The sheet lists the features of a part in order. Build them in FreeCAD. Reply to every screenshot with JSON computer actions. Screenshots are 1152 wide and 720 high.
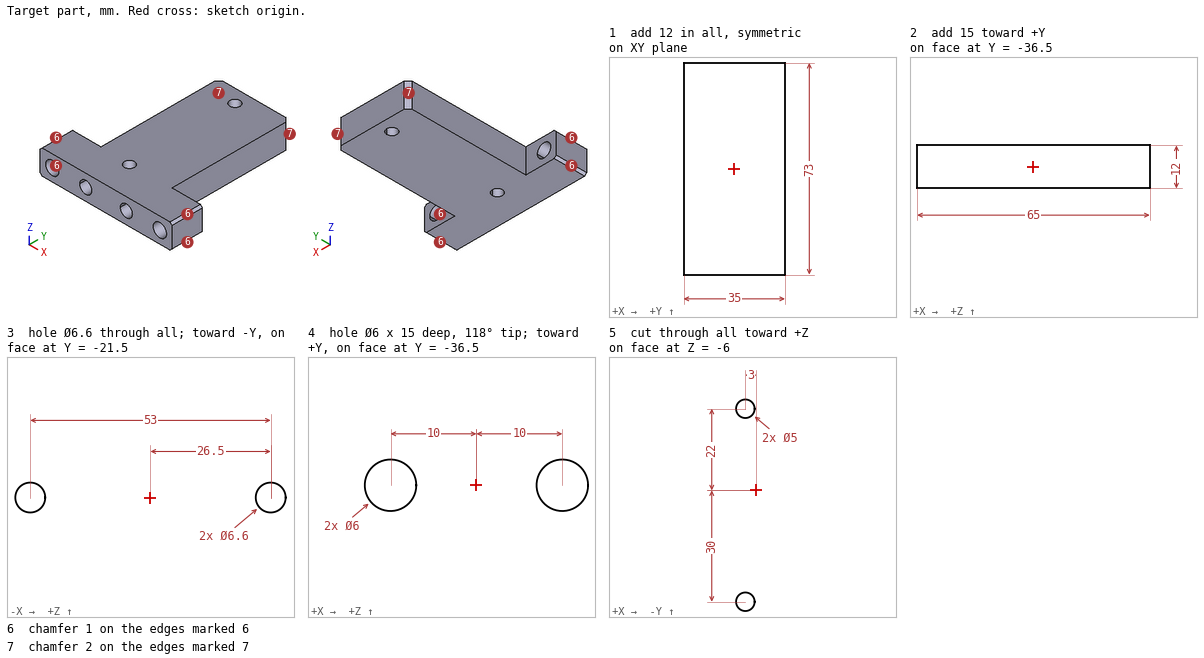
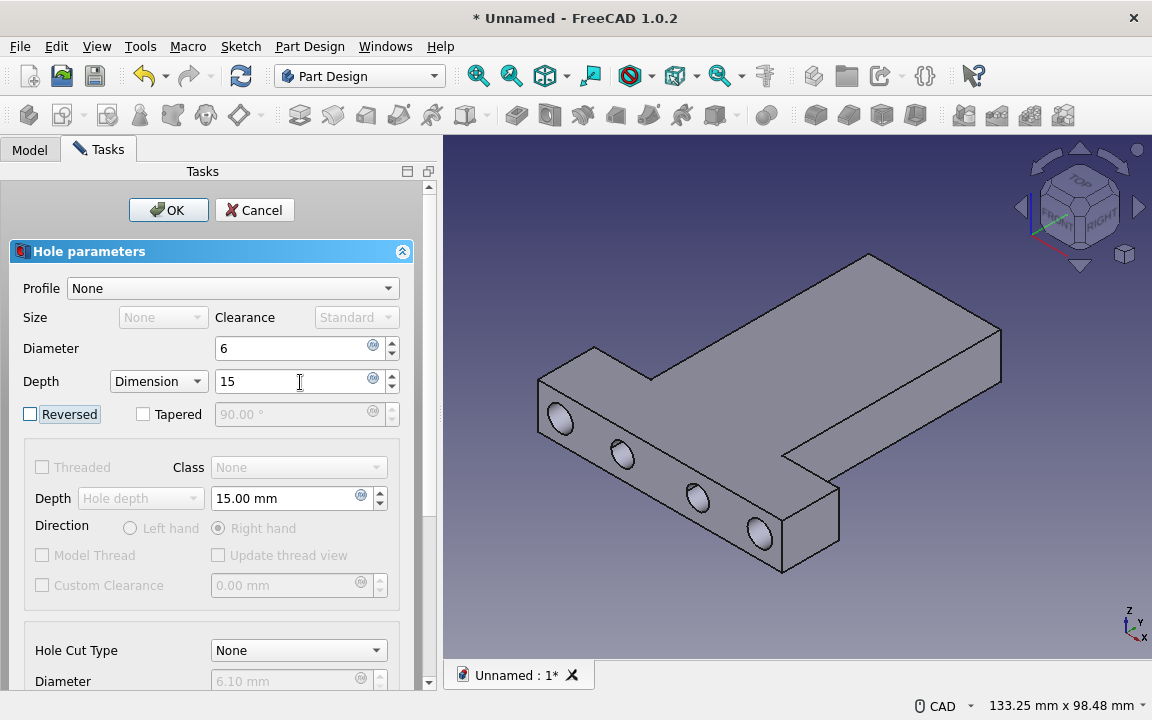
{"action": "left_click", "coordinate": [169, 210]}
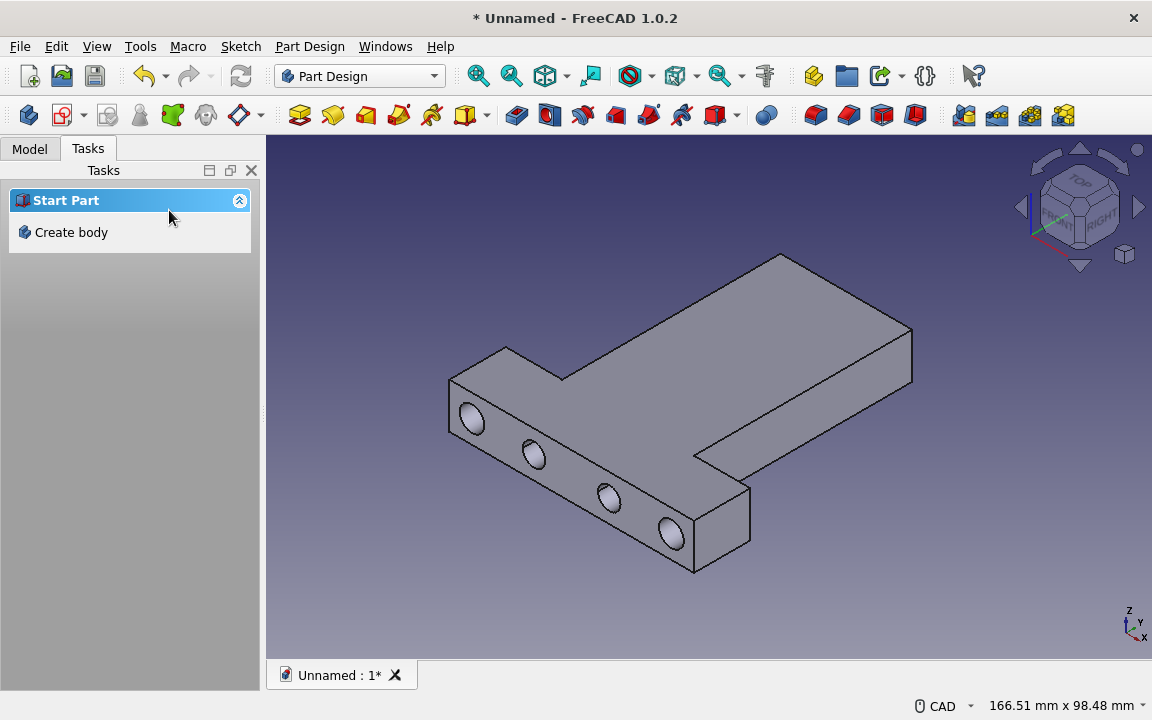
{"action": "key", "text": "5"}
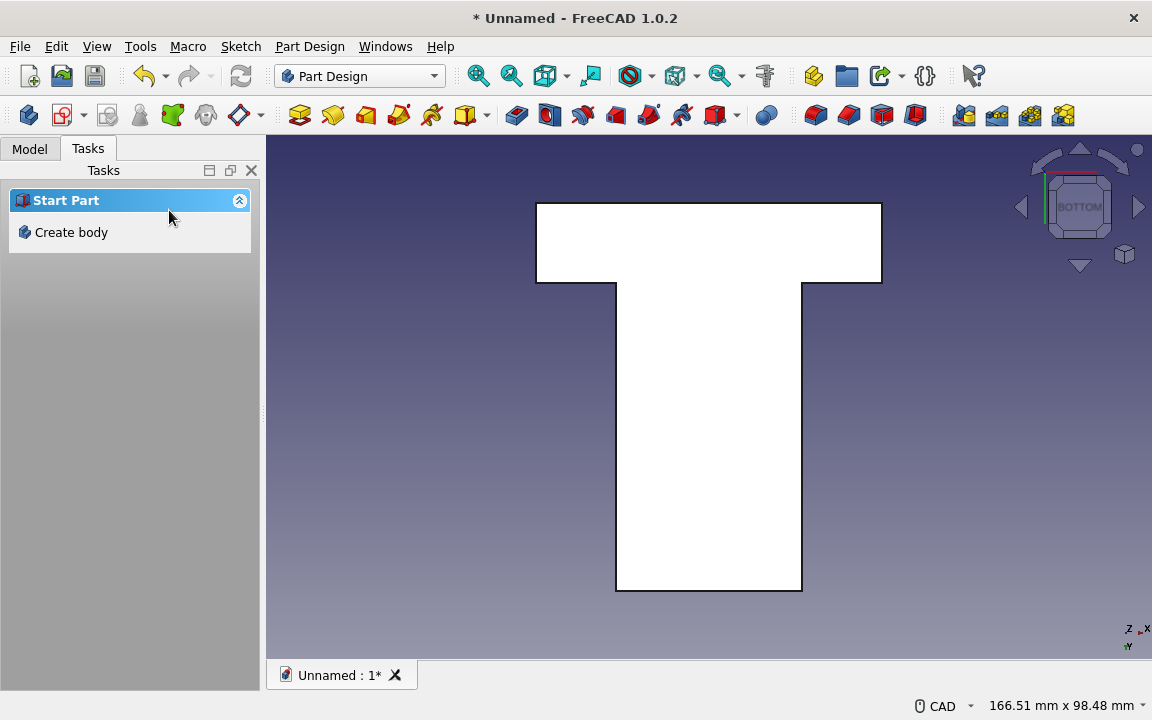
{"action": "left_click", "coordinate": [709, 451]}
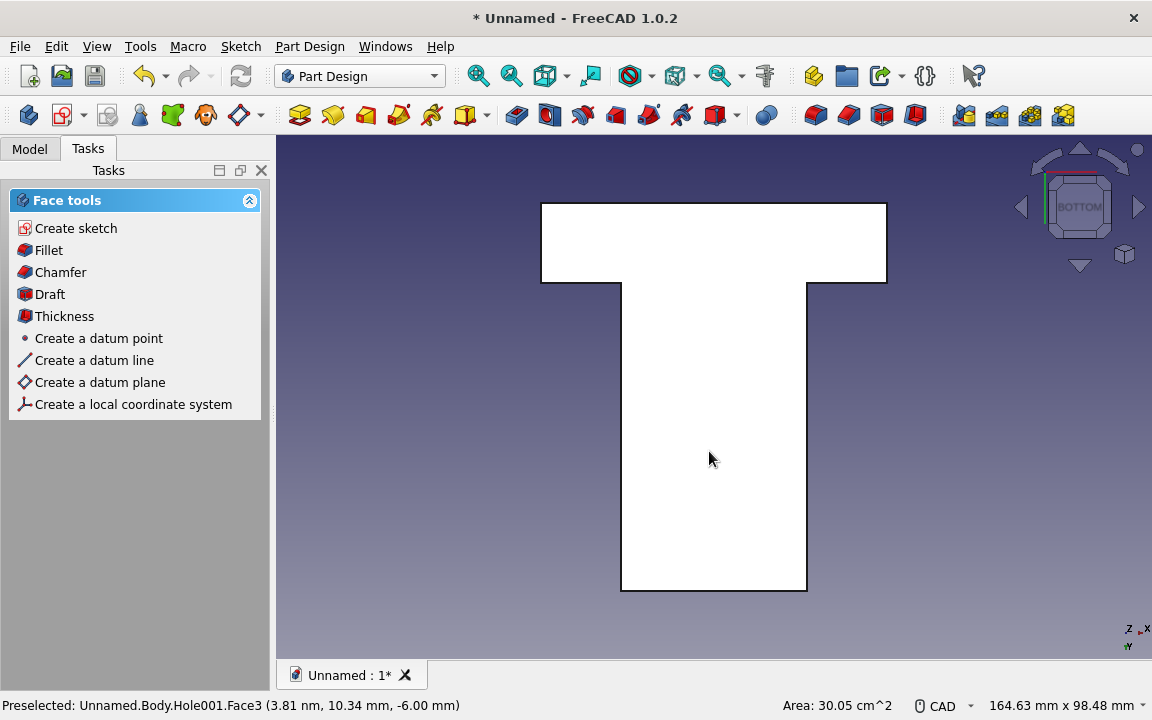
{"action": "left_click", "coordinate": [62, 116]}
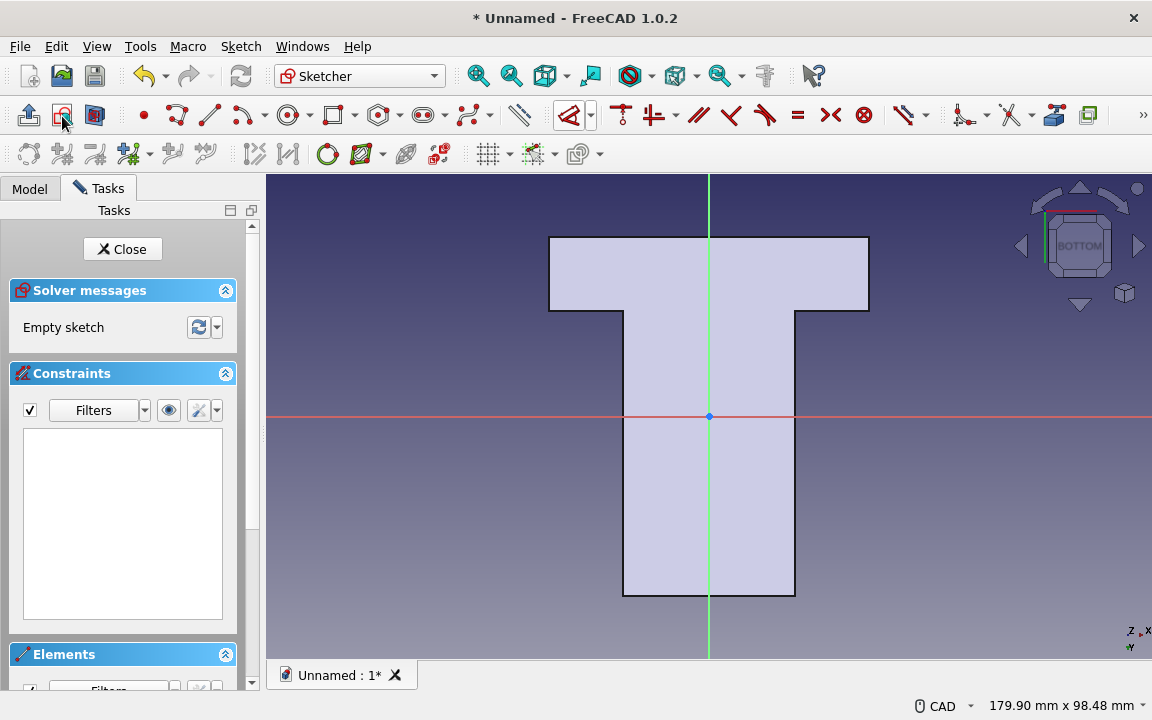
{"action": "left_click", "coordinate": [288, 116]}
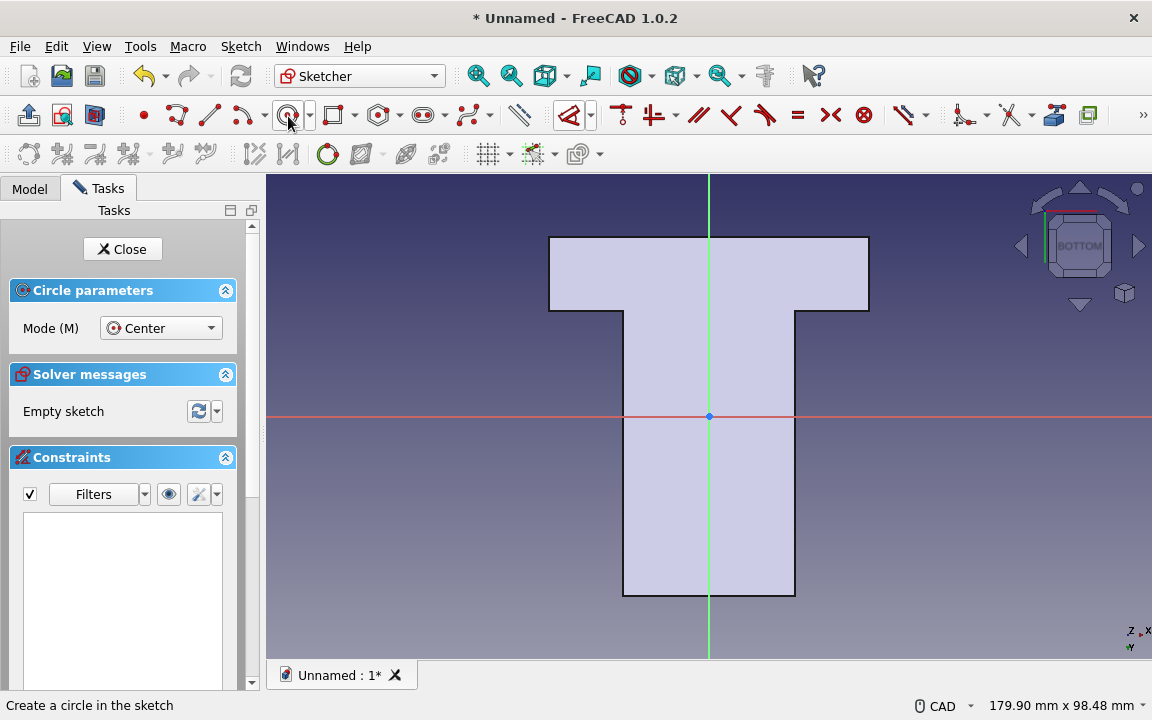
{"action": "scroll", "coordinate": [694, 308], "scroll_direction": "up", "scroll_amount": 4}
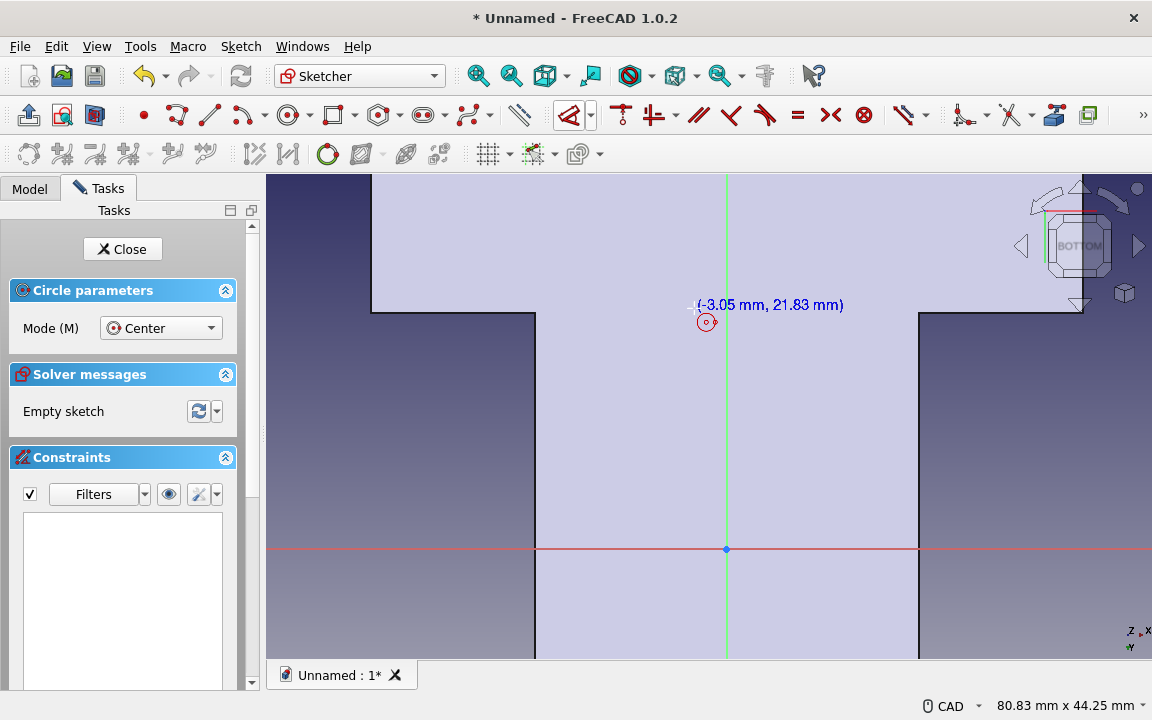
{"action": "left_click", "coordinate": [694, 308]}
{"action": "mouse_move", "coordinate": [675, 289]}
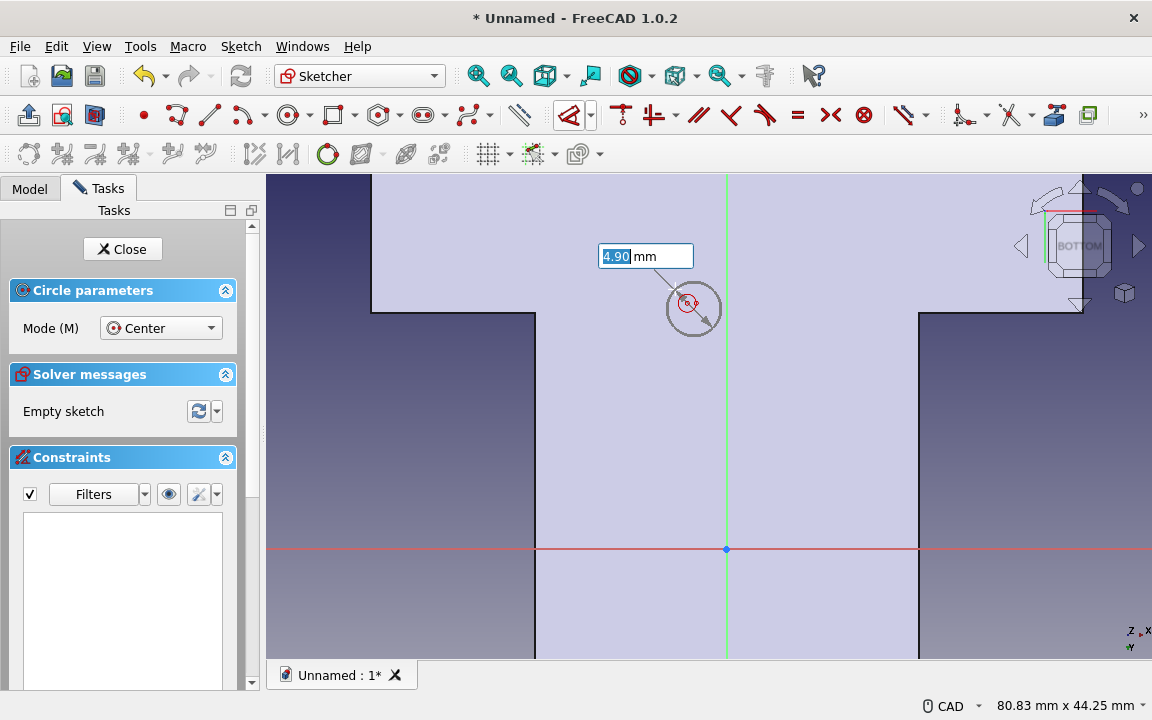
{"action": "type", "text": "5"}
{"action": "key", "text": "Return"}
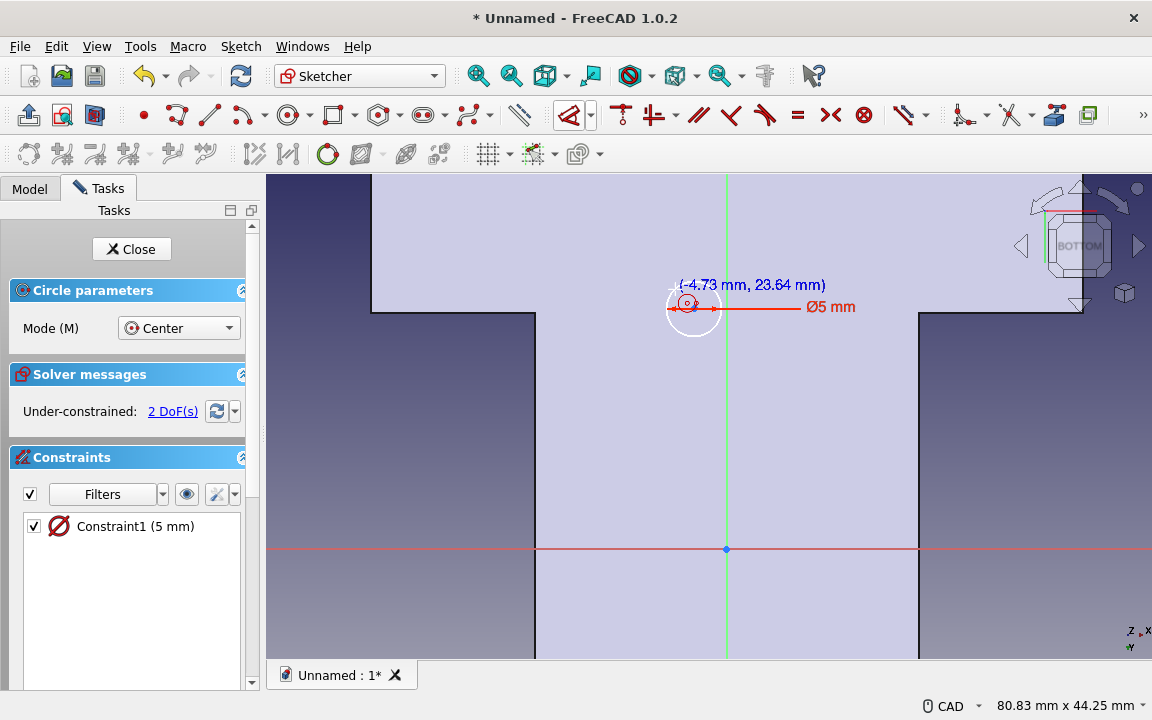
{"action": "scroll", "coordinate": [595, 273], "scroll_direction": "down", "scroll_amount": 4}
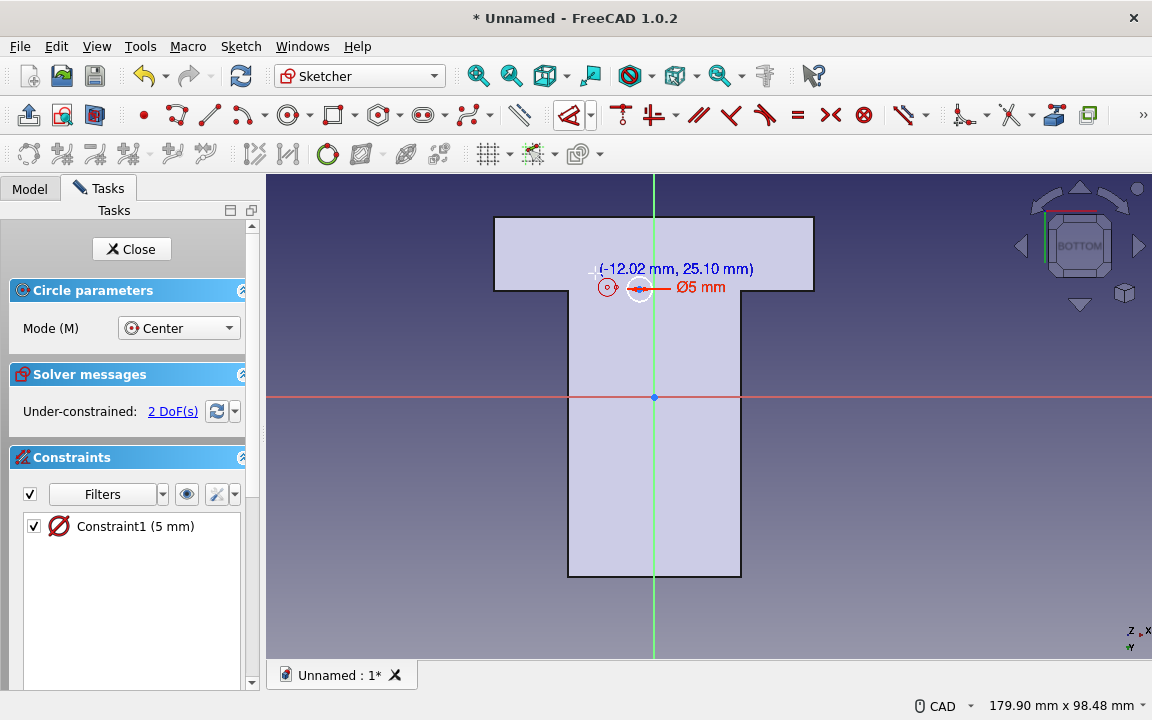
{"action": "scroll", "coordinate": [640, 545], "scroll_direction": "up", "scroll_amount": 4}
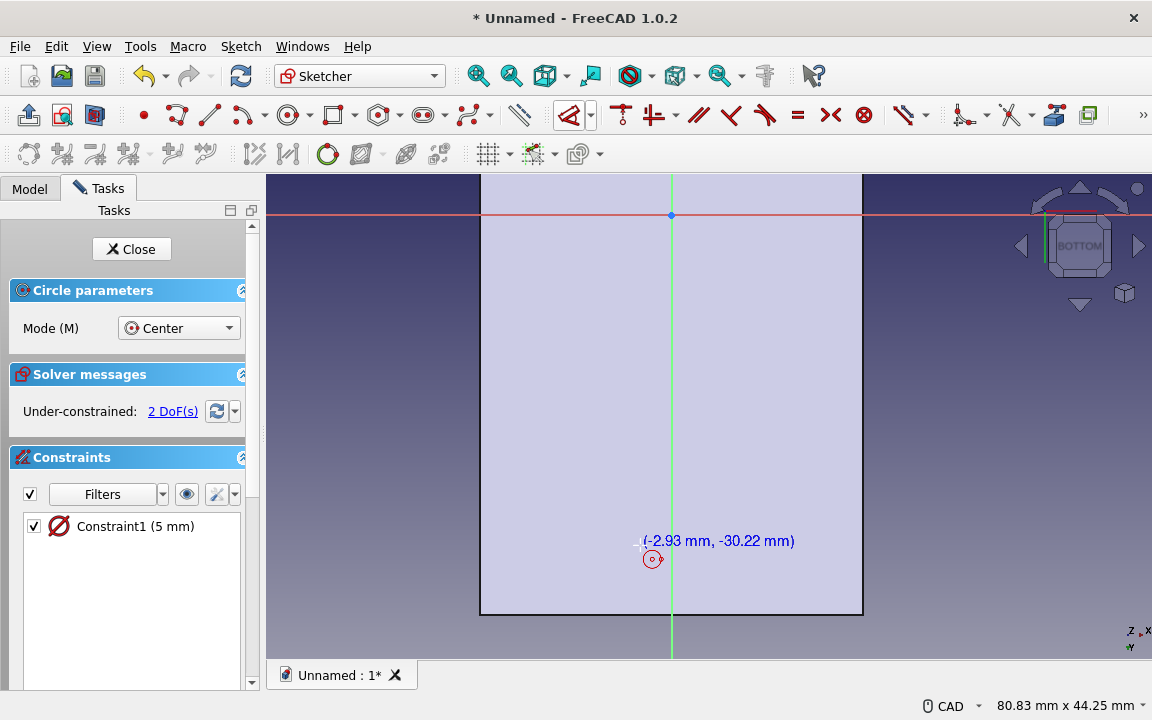
{"action": "left_click", "coordinate": [639, 544]}
{"action": "mouse_move", "coordinate": [619, 525]}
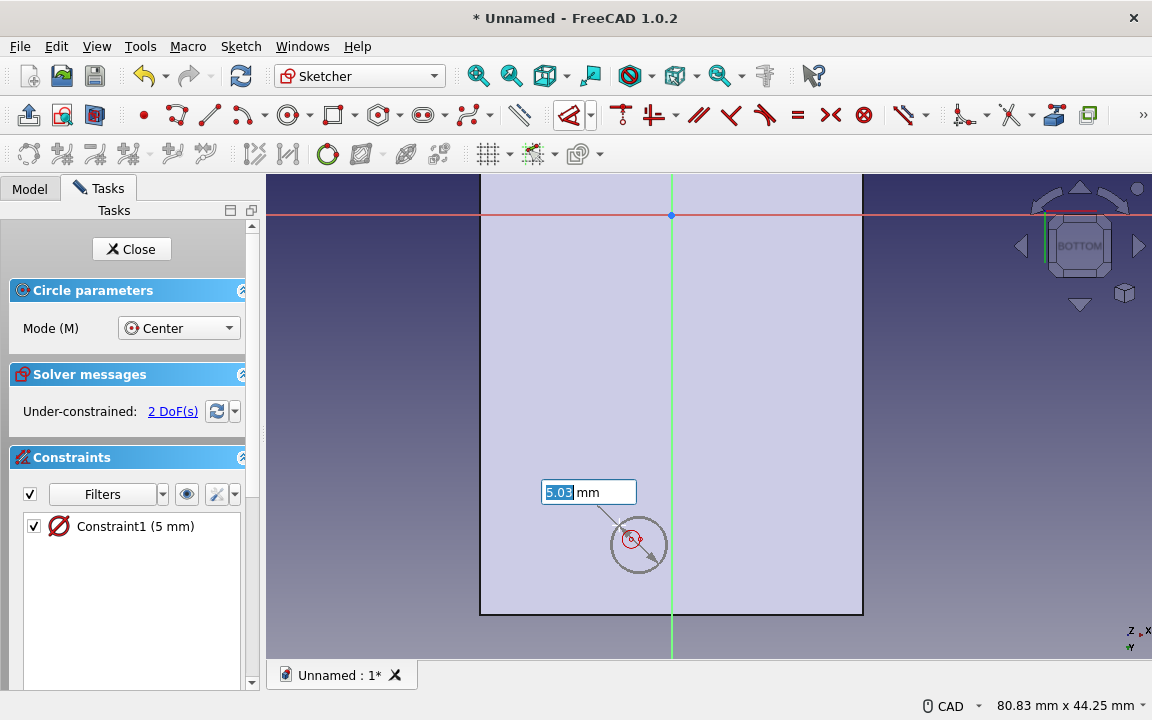
{"action": "type", "text": "5"}
{"action": "key", "text": "Return"}
{"action": "key", "text": "Escape"}